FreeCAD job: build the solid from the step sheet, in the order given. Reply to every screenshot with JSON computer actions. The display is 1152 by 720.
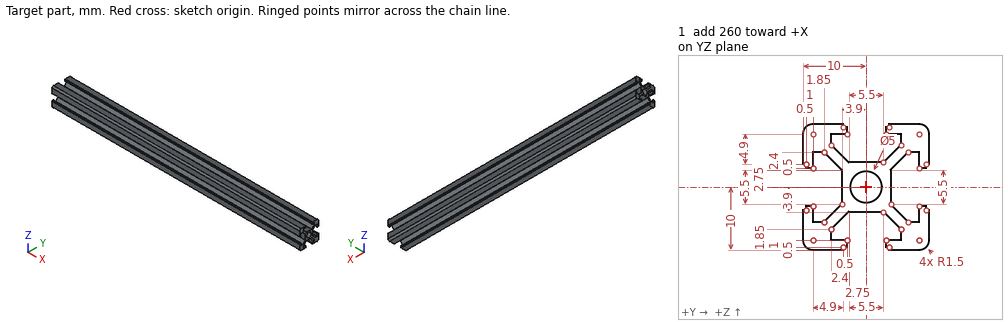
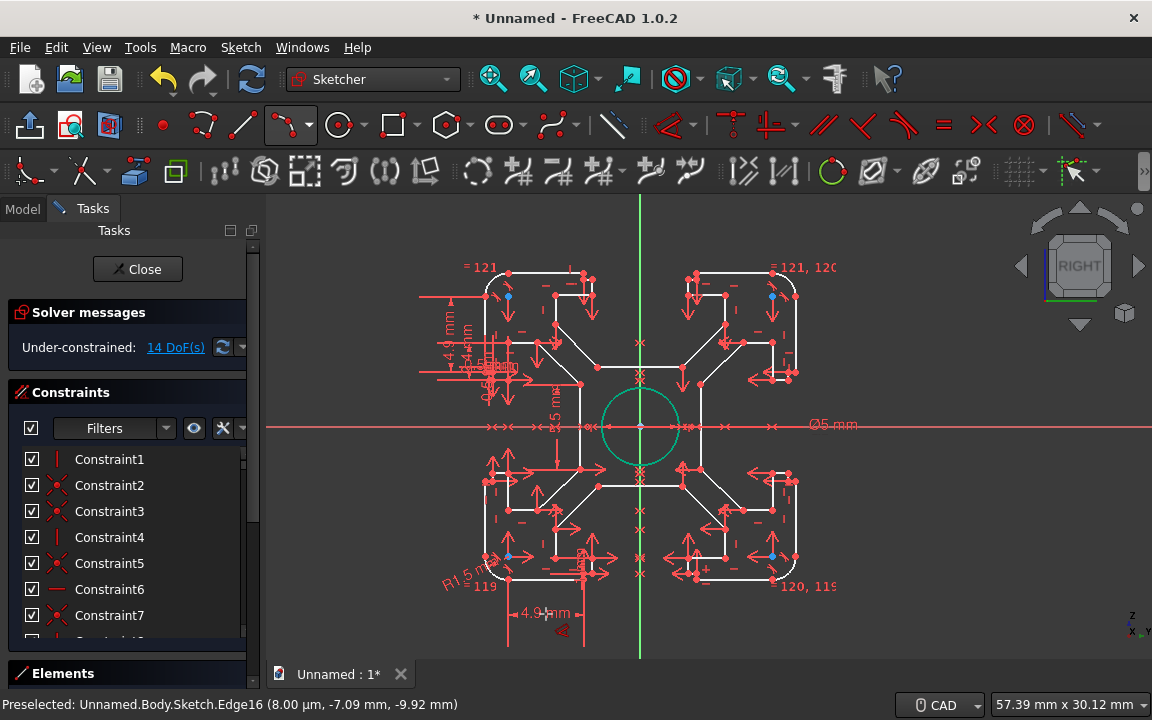
{"action": "scroll", "coordinate": [584, 577], "scroll_direction": "up", "scroll_amount": 9}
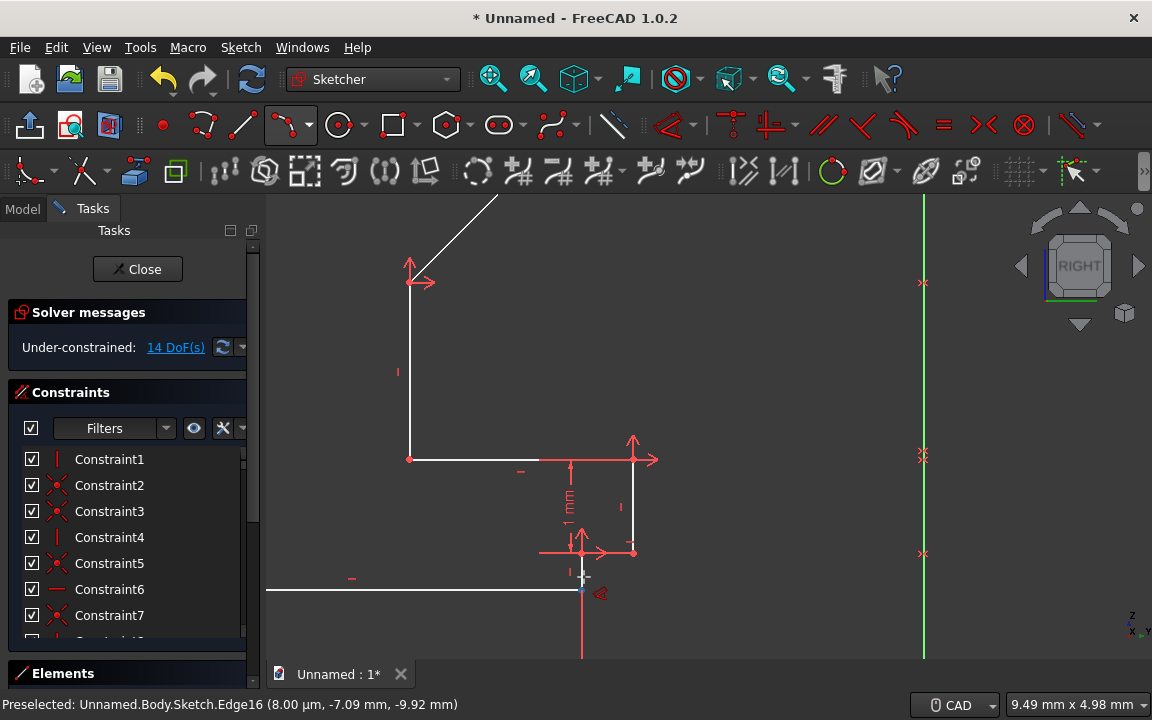
{"action": "left_click", "coordinate": [582, 572]}
{"action": "left_click", "coordinate": [548, 572]}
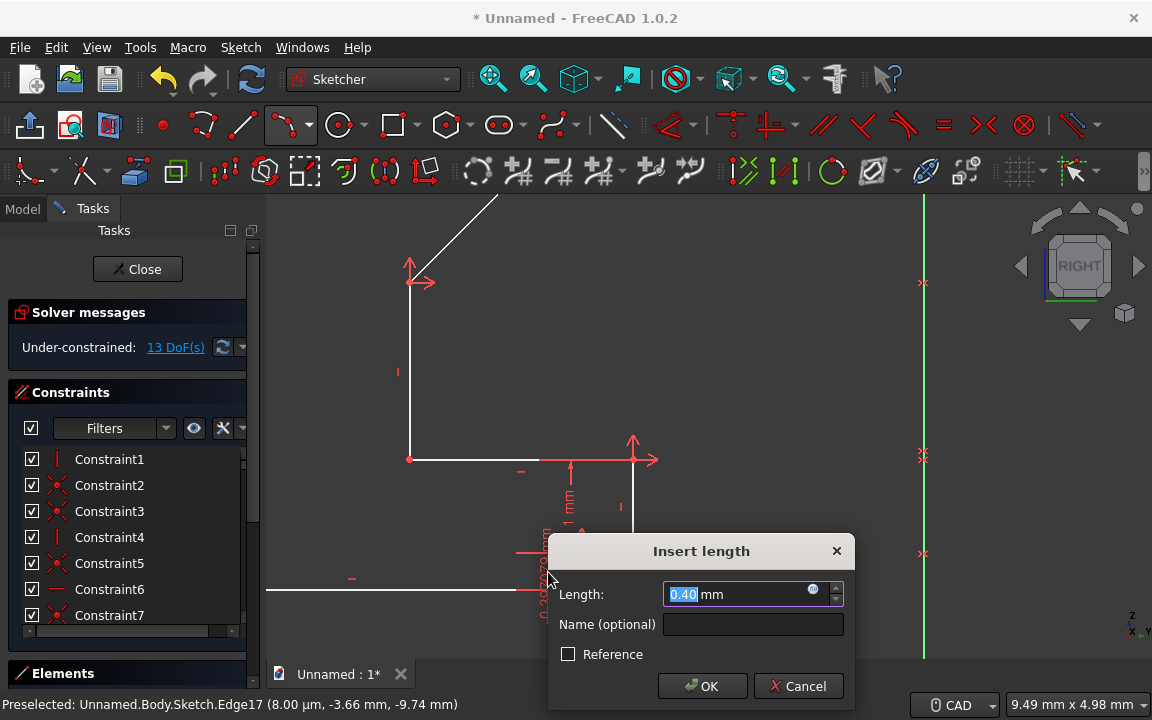
{"action": "type", "text": "0.5"}
{"action": "key", "text": "Return"}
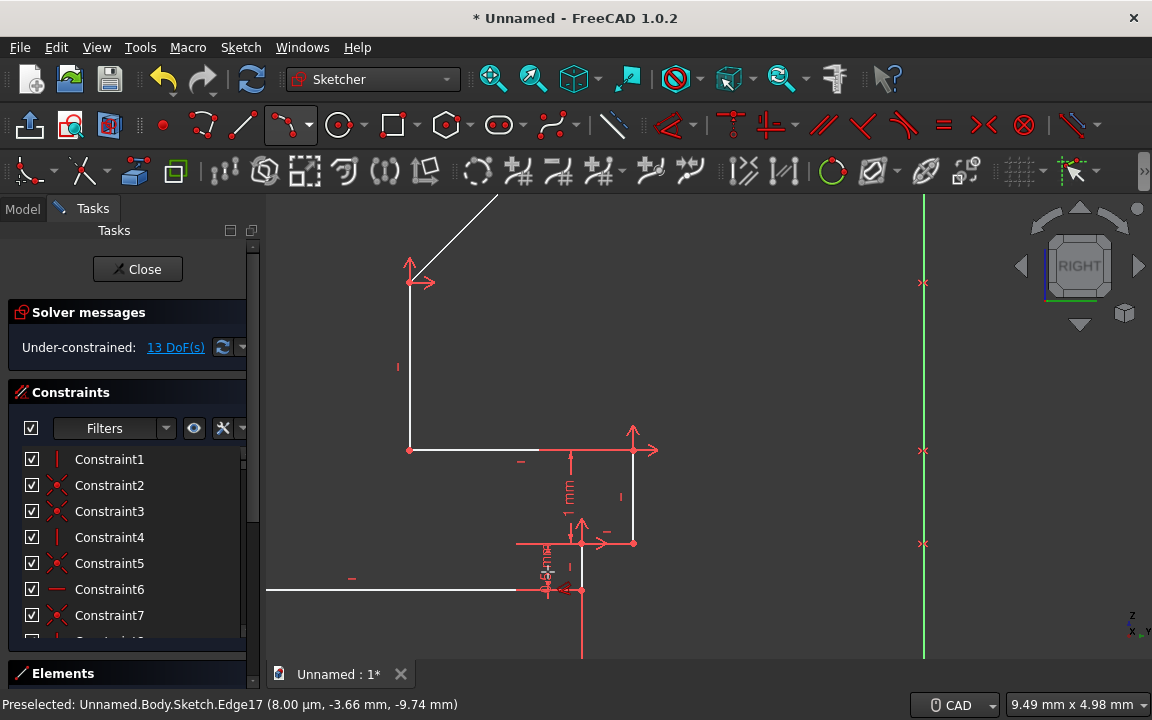
{"action": "left_click", "coordinate": [597, 544]}
{"action": "left_click", "coordinate": [619, 578]}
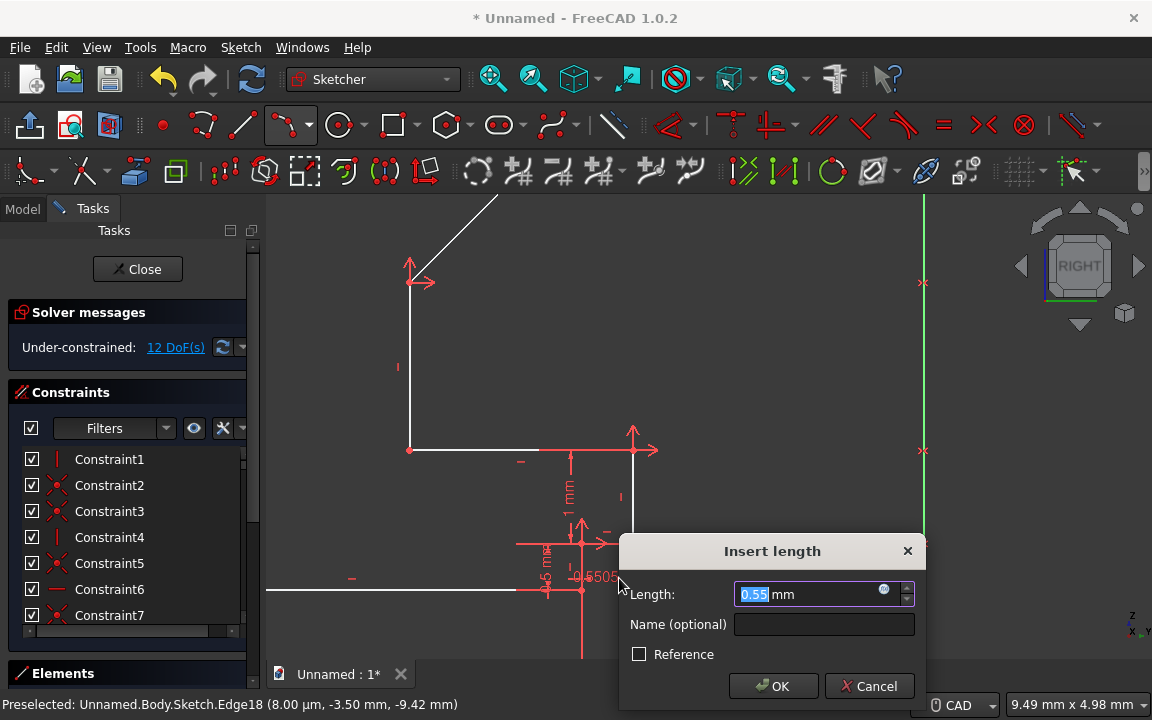
{"action": "type", "text": "0.5"}
{"action": "key", "text": "Return"}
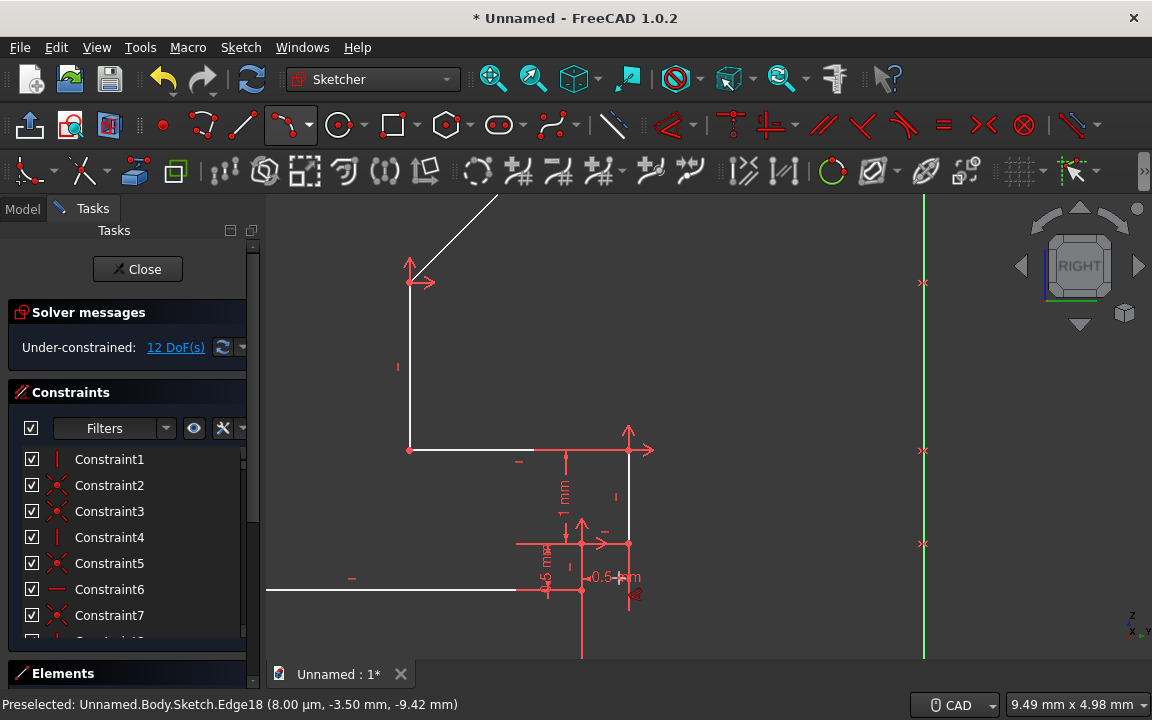
{"action": "scroll", "coordinate": [584, 578], "scroll_direction": "down", "scroll_amount": 9}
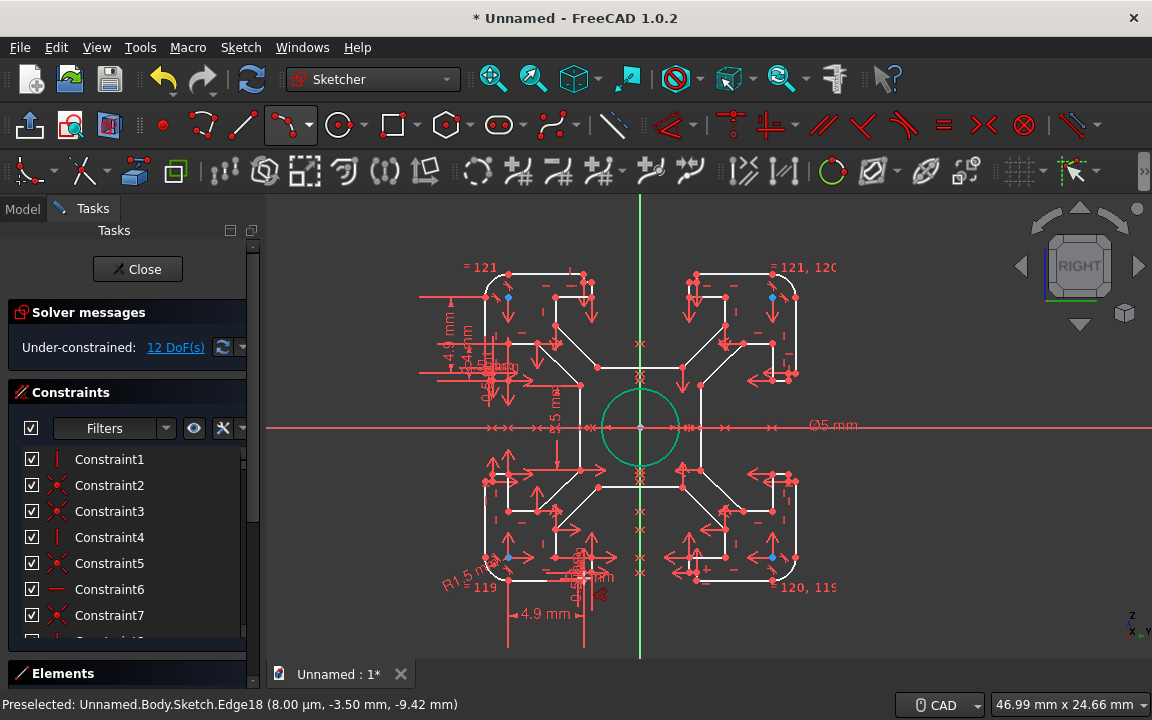
{"action": "scroll", "coordinate": [581, 558], "scroll_direction": "up", "scroll_amount": 2}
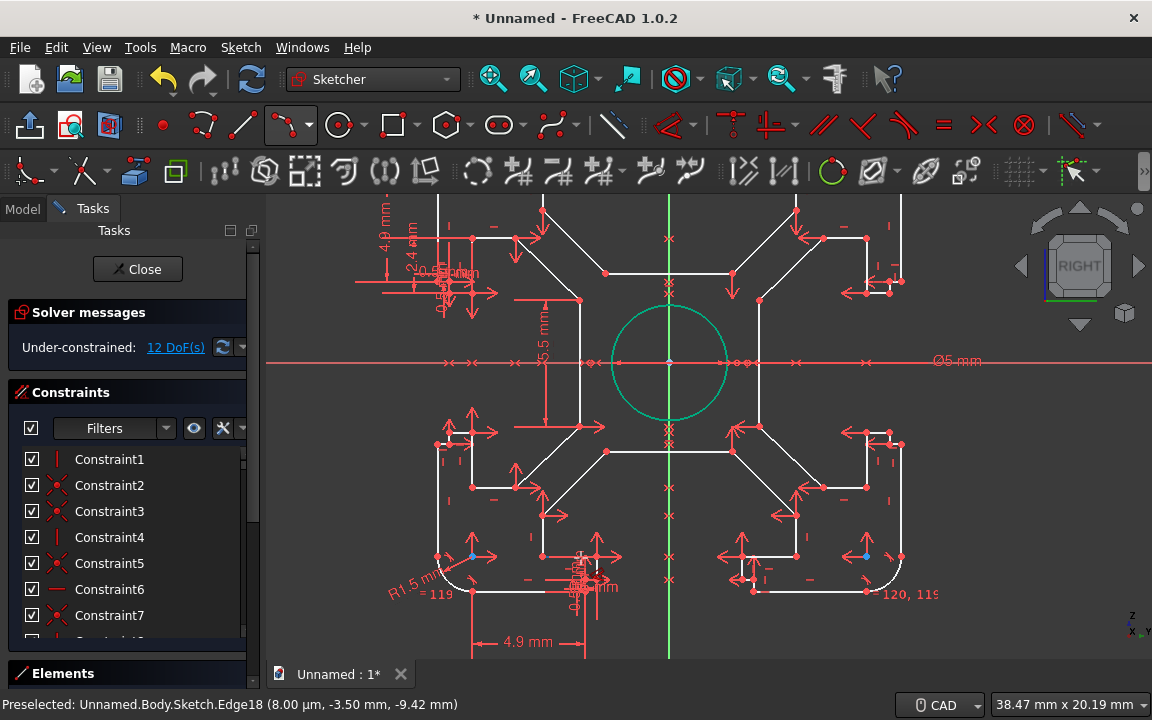
{"action": "left_click", "coordinate": [581, 557]}
{"action": "left_click", "coordinate": [570, 523]}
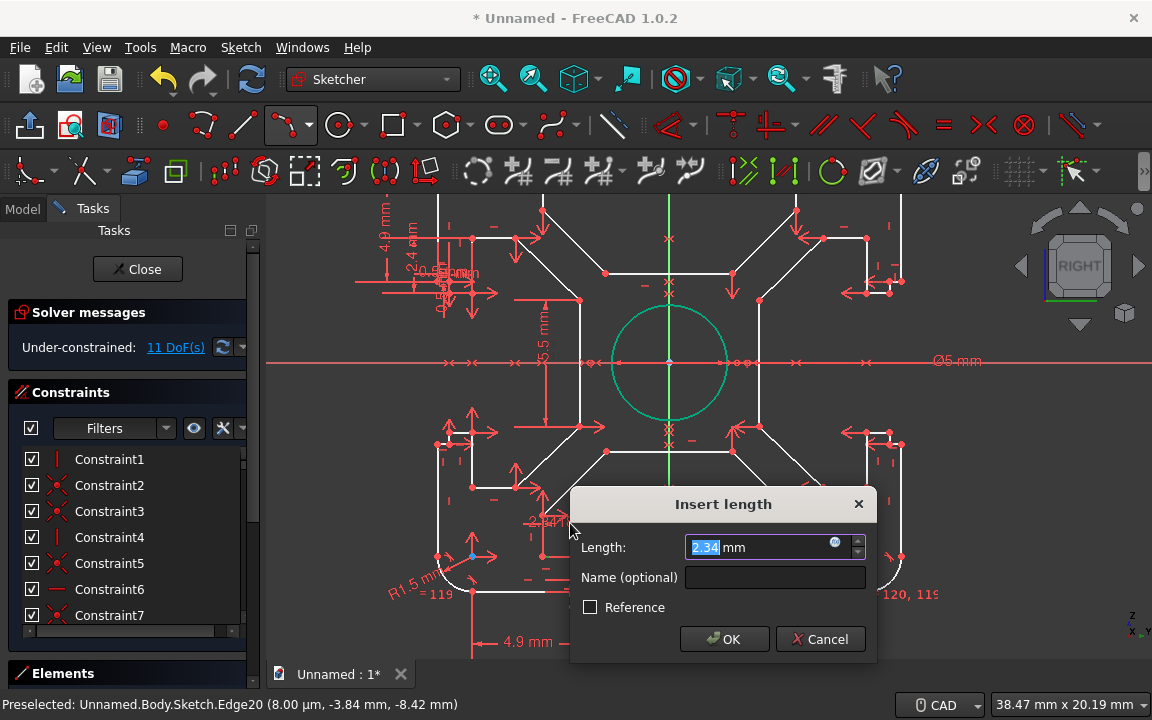
{"action": "type", "text": "2.4"}
{"action": "key", "text": "Return"}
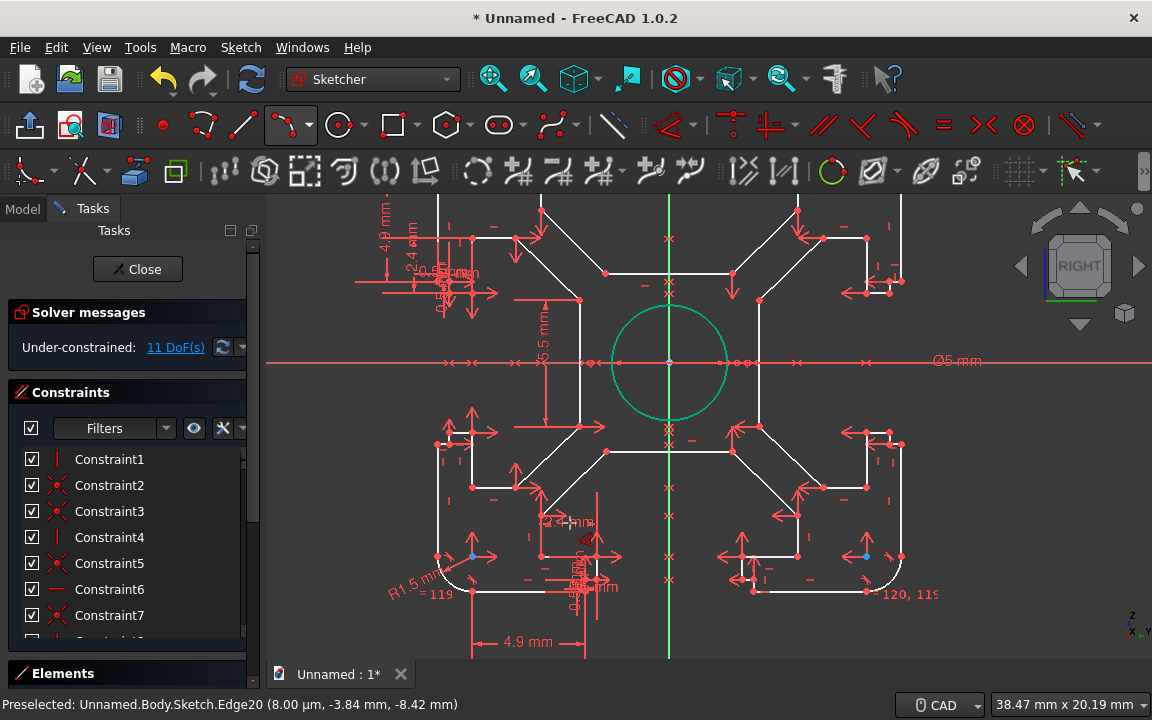
{"action": "left_click", "coordinate": [644, 452]}
{"action": "left_click", "coordinate": [641, 486]}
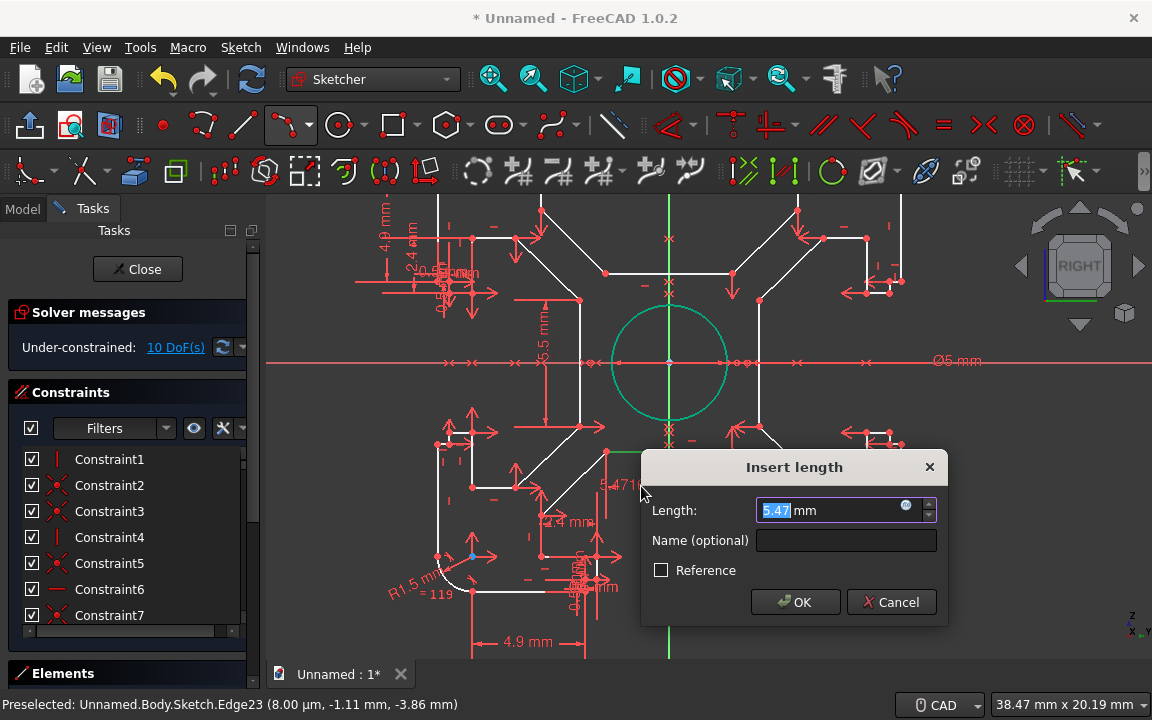
{"action": "type", "text": "5.5"}
{"action": "key", "text": "Return"}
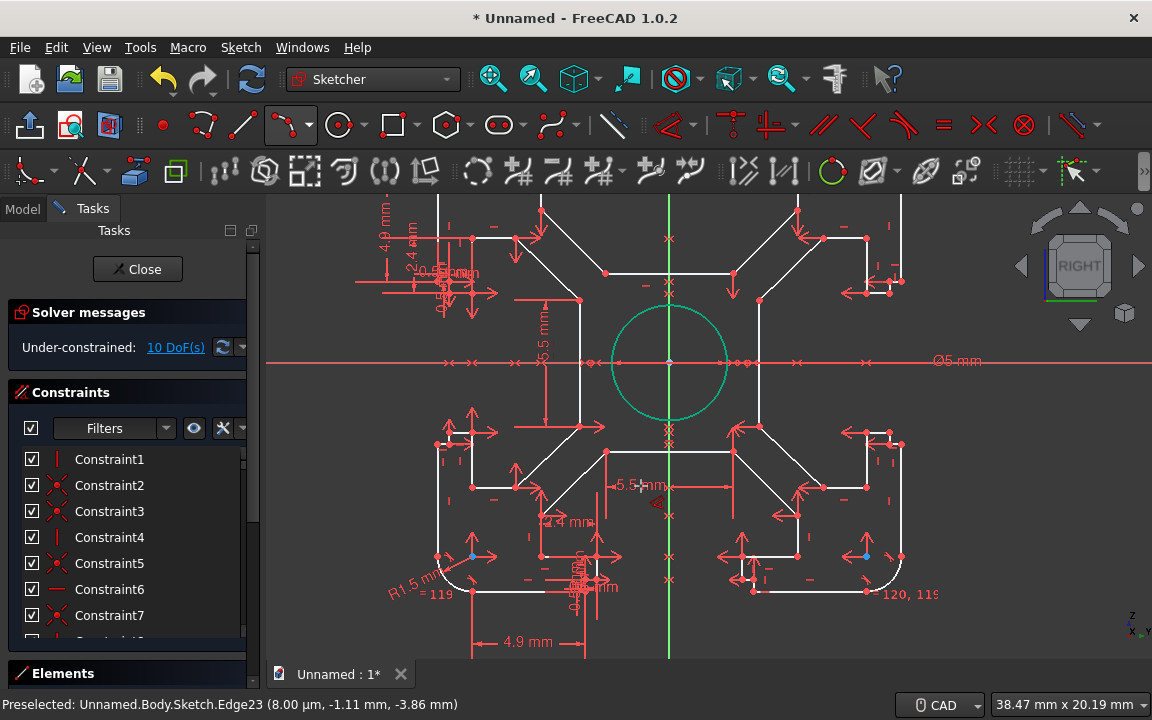
{"action": "left_click", "coordinate": [759, 389]}
{"action": "left_click", "coordinate": [793, 335]}